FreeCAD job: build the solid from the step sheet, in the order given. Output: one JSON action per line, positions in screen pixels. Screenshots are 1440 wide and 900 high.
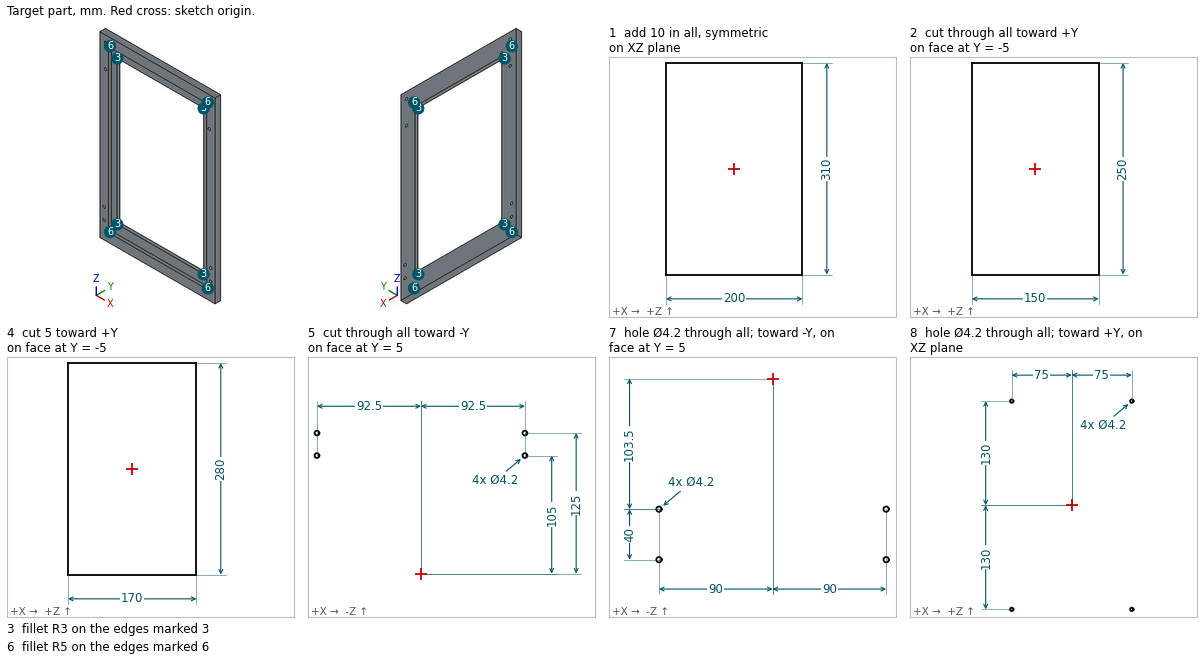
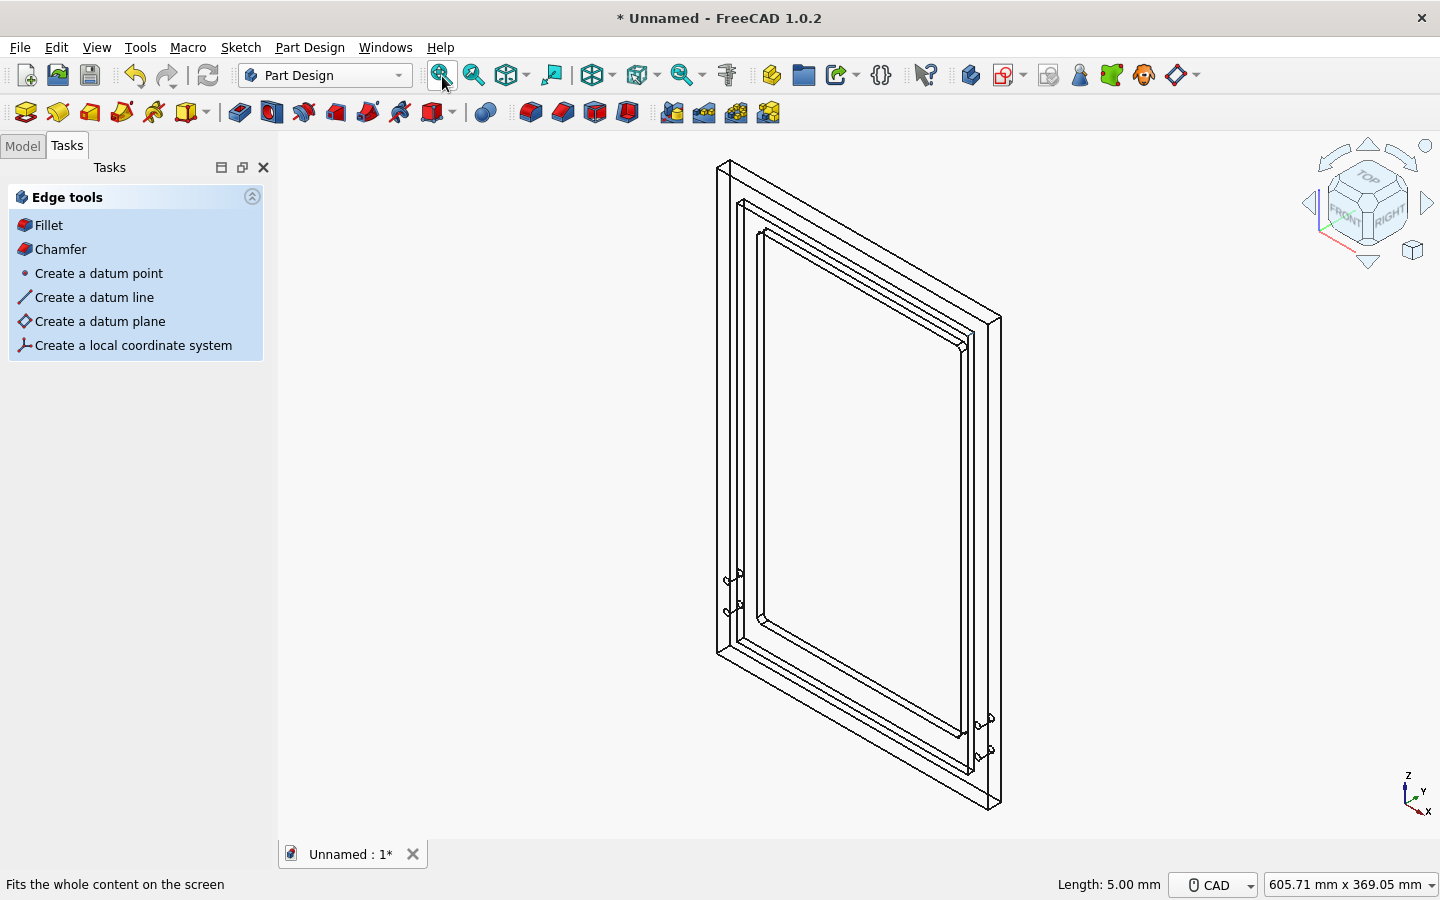
{"action": "key", "text": "2"}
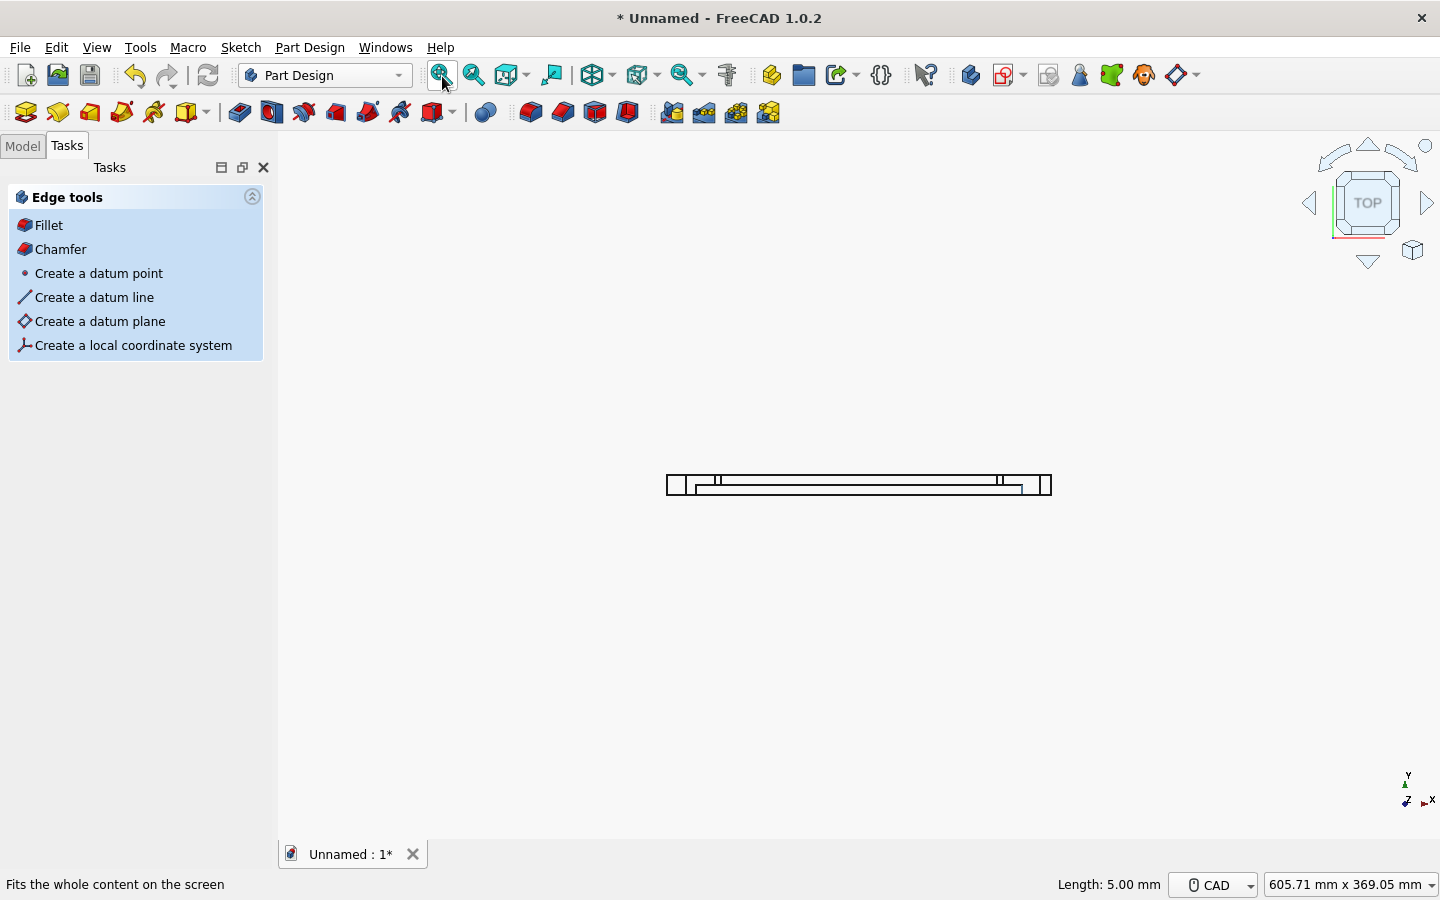
{"action": "key", "text": "v f"}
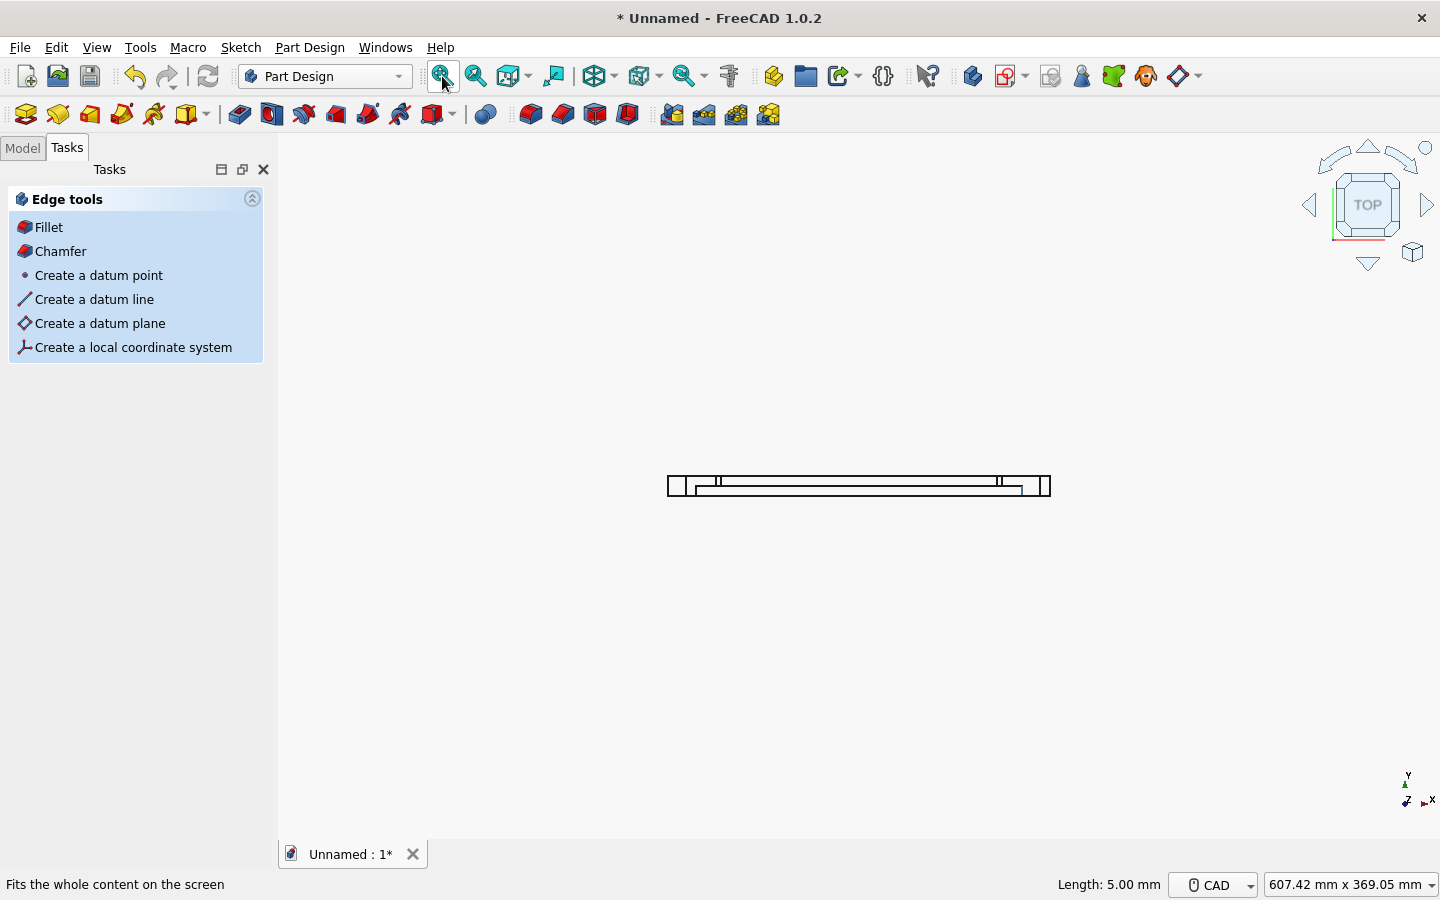
{"action": "scroll", "coordinate": [1022, 490], "scroll_direction": "up", "scroll_amount": 8}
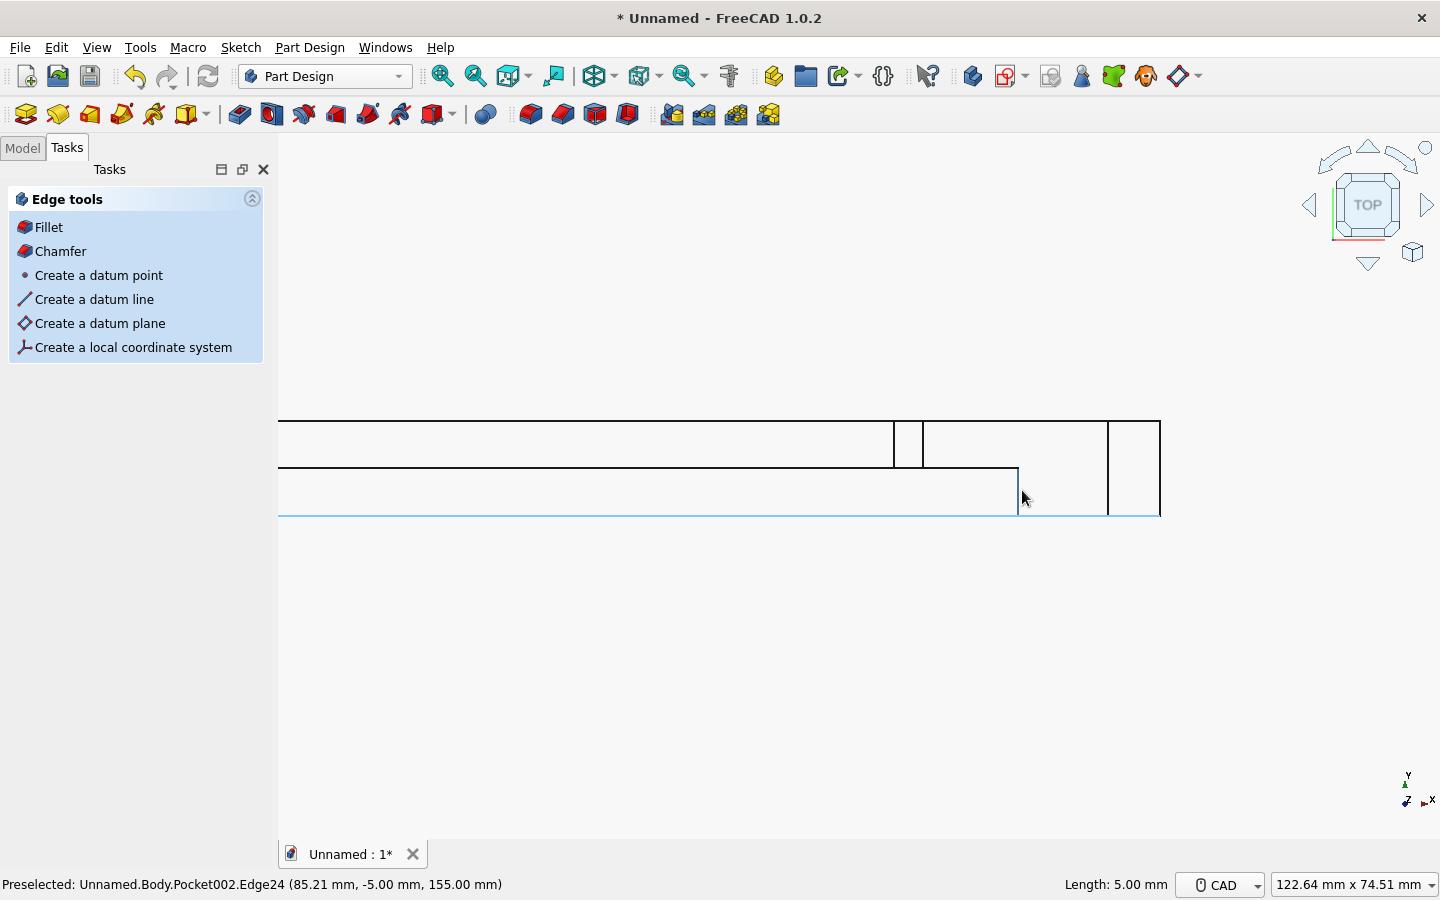
{"action": "key", "text": "v f"}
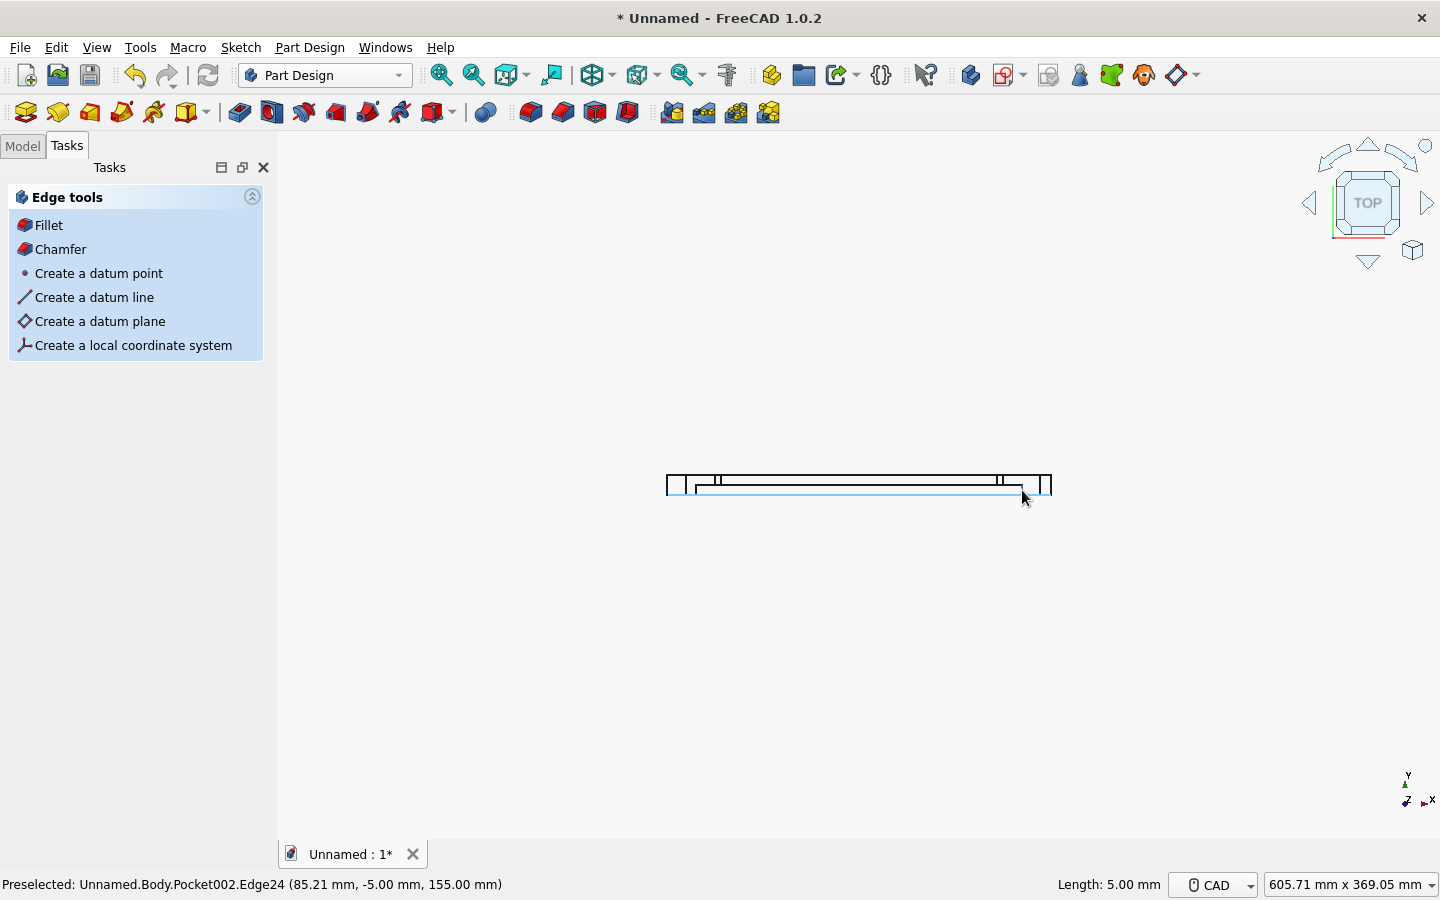
{"action": "key", "text": "1"}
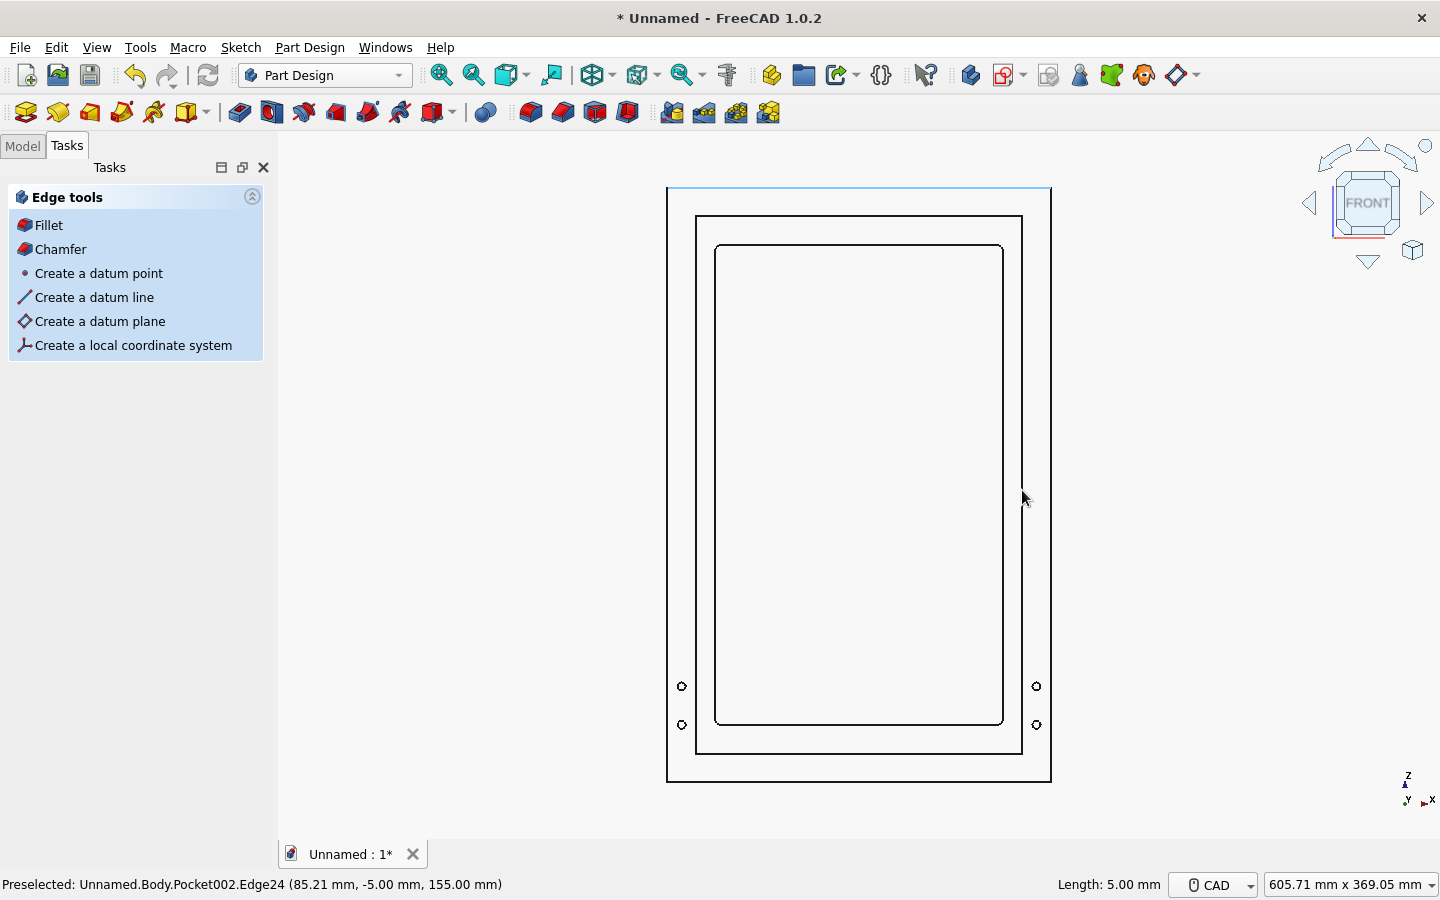
{"action": "scroll", "coordinate": [1022, 753], "scroll_direction": "up", "scroll_amount": 8}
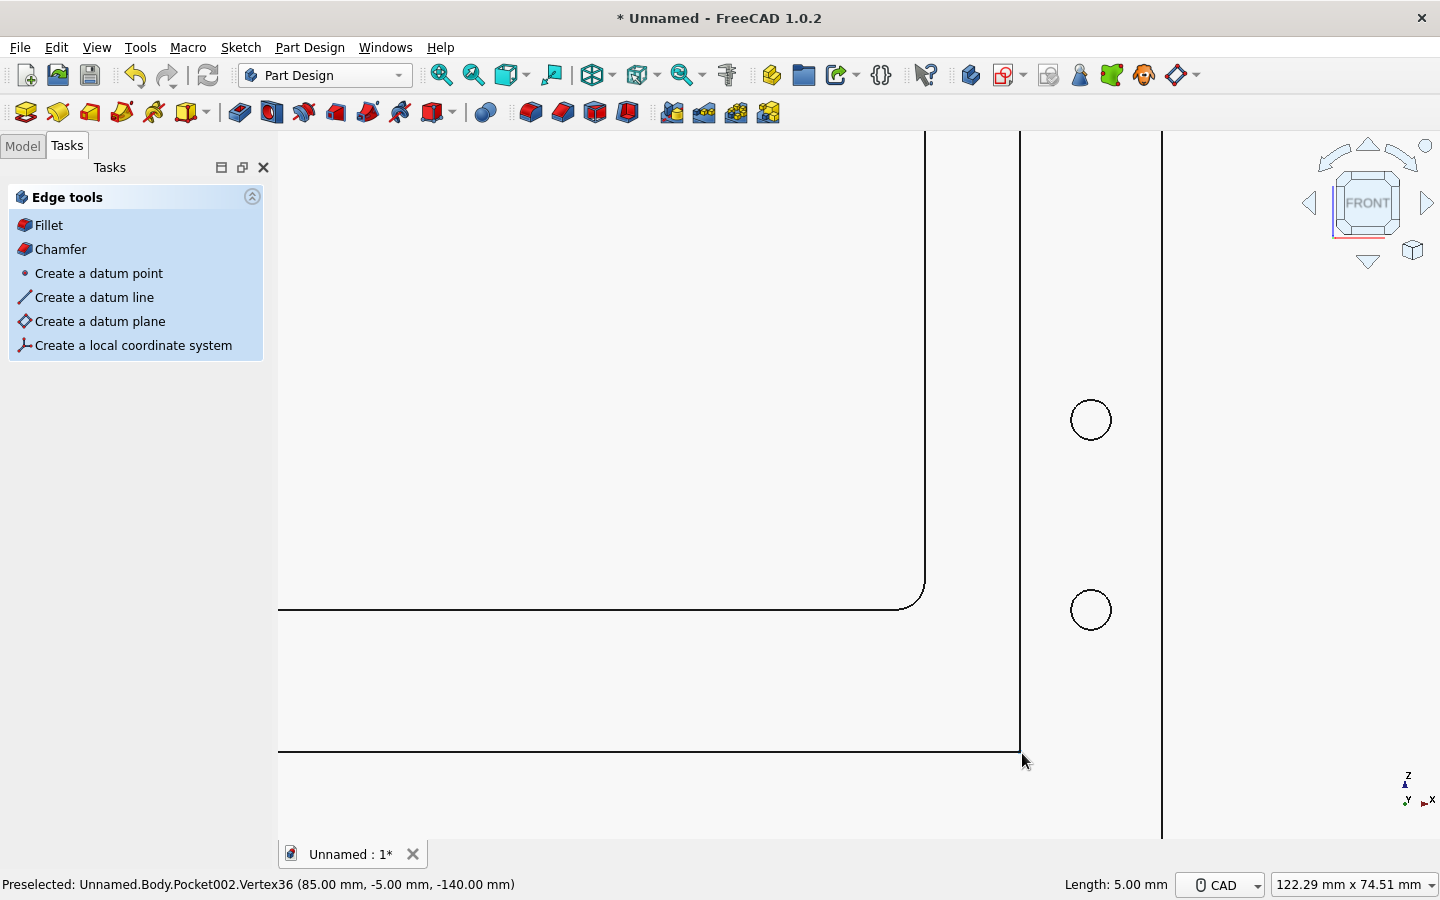
{"action": "key", "text": "v f"}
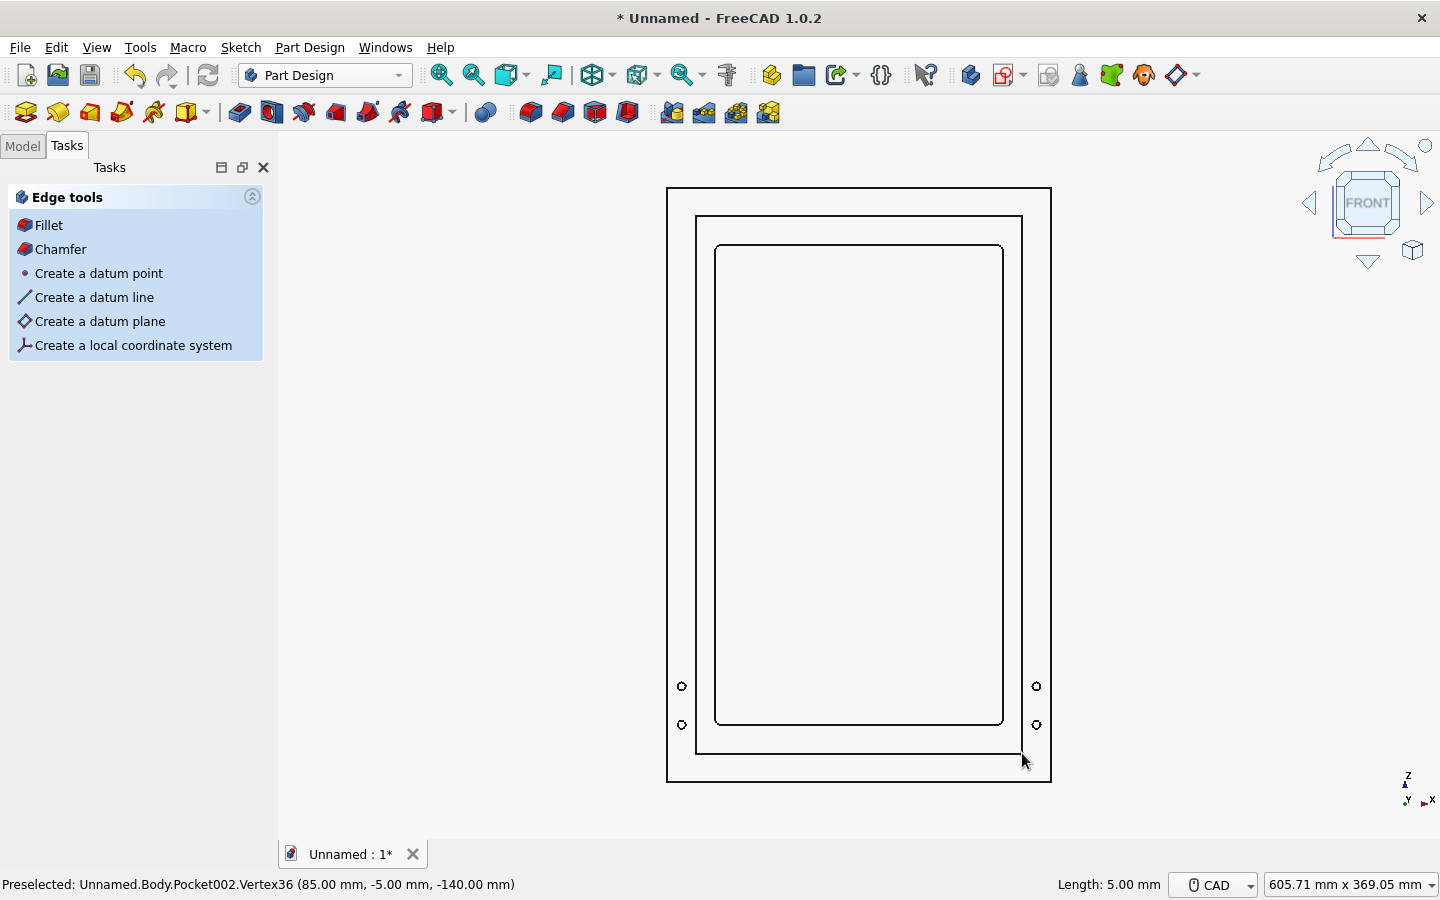
{"action": "key", "text": "3"}